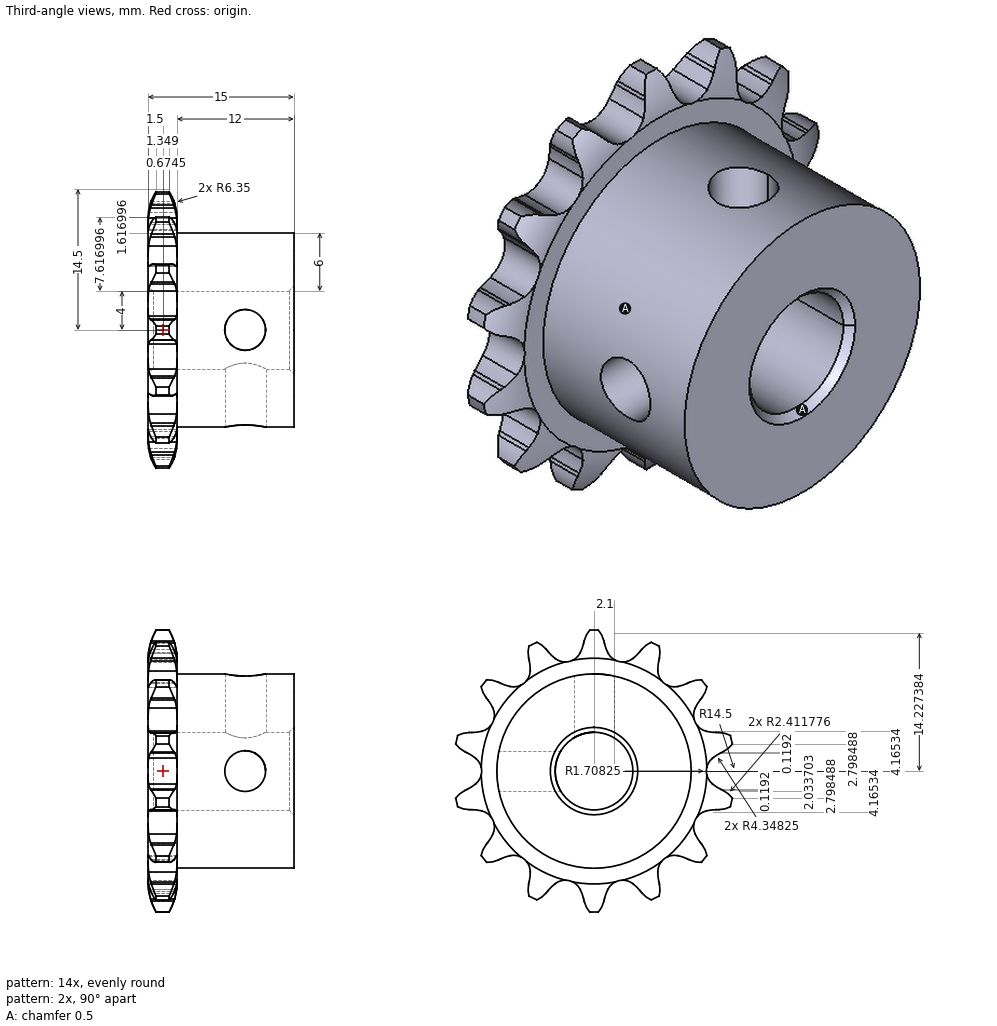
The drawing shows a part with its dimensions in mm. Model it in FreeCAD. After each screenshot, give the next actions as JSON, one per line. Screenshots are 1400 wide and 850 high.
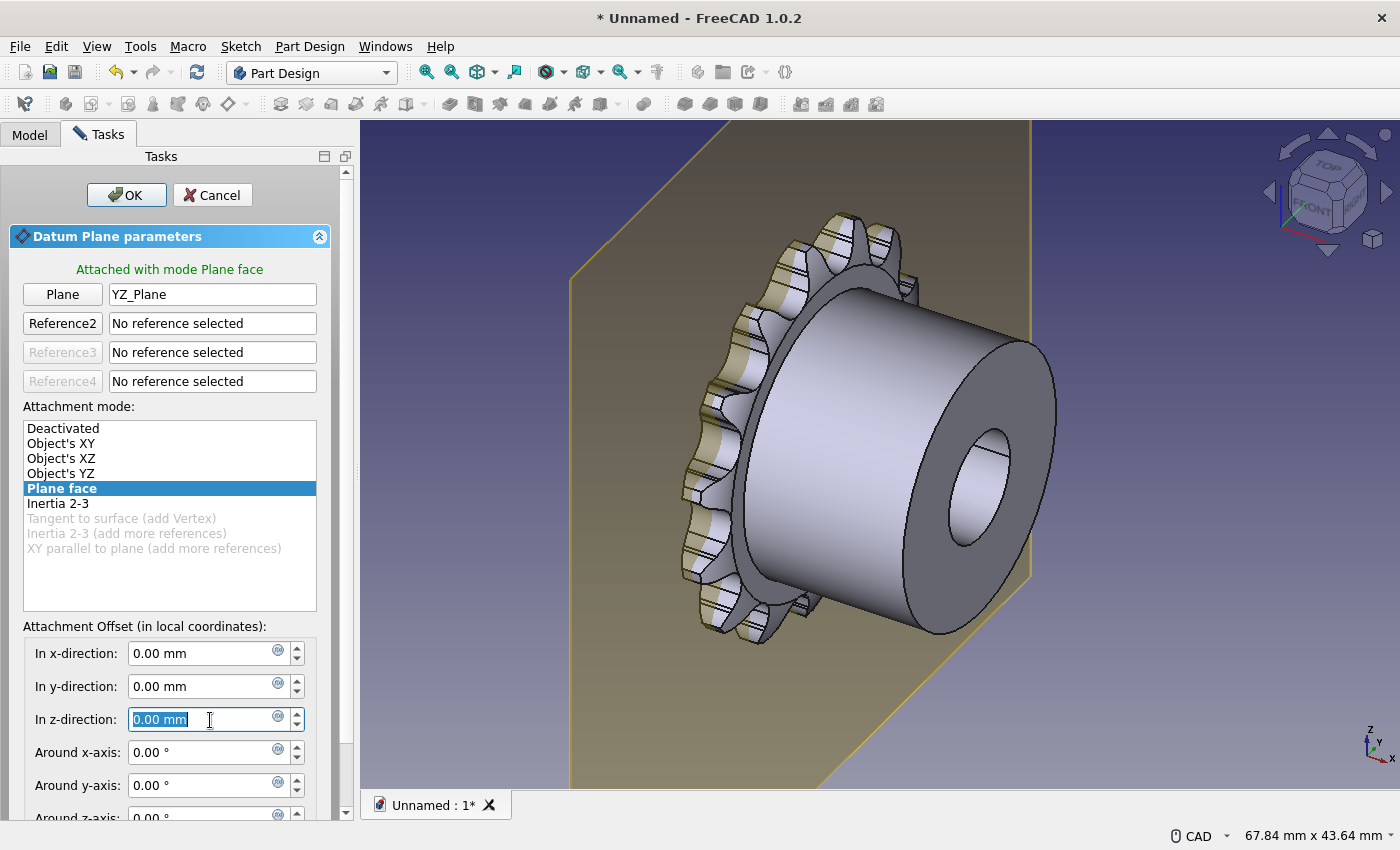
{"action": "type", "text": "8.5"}
{"action": "key", "text": "Tab"}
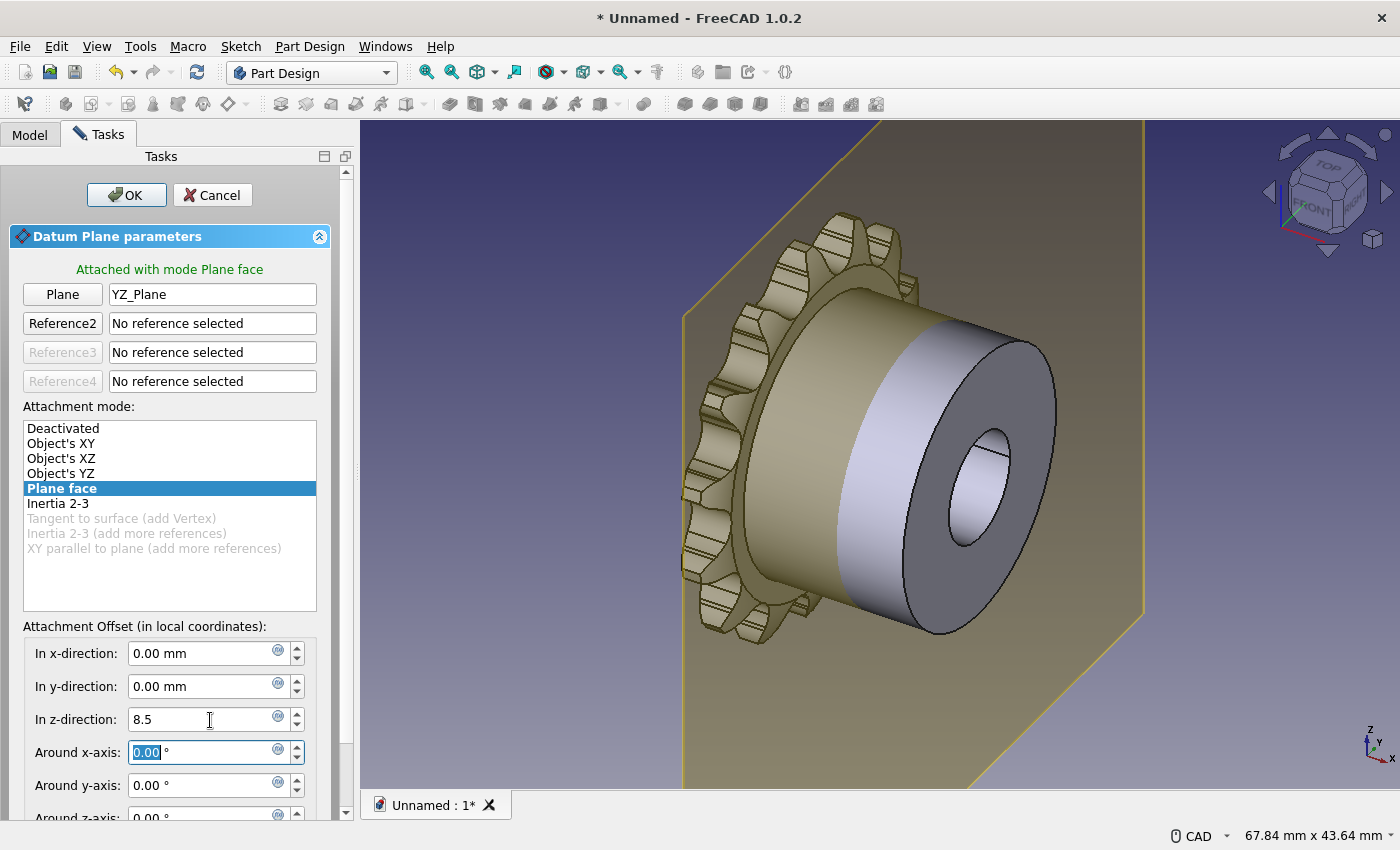
{"action": "left_click", "coordinate": [127, 195]}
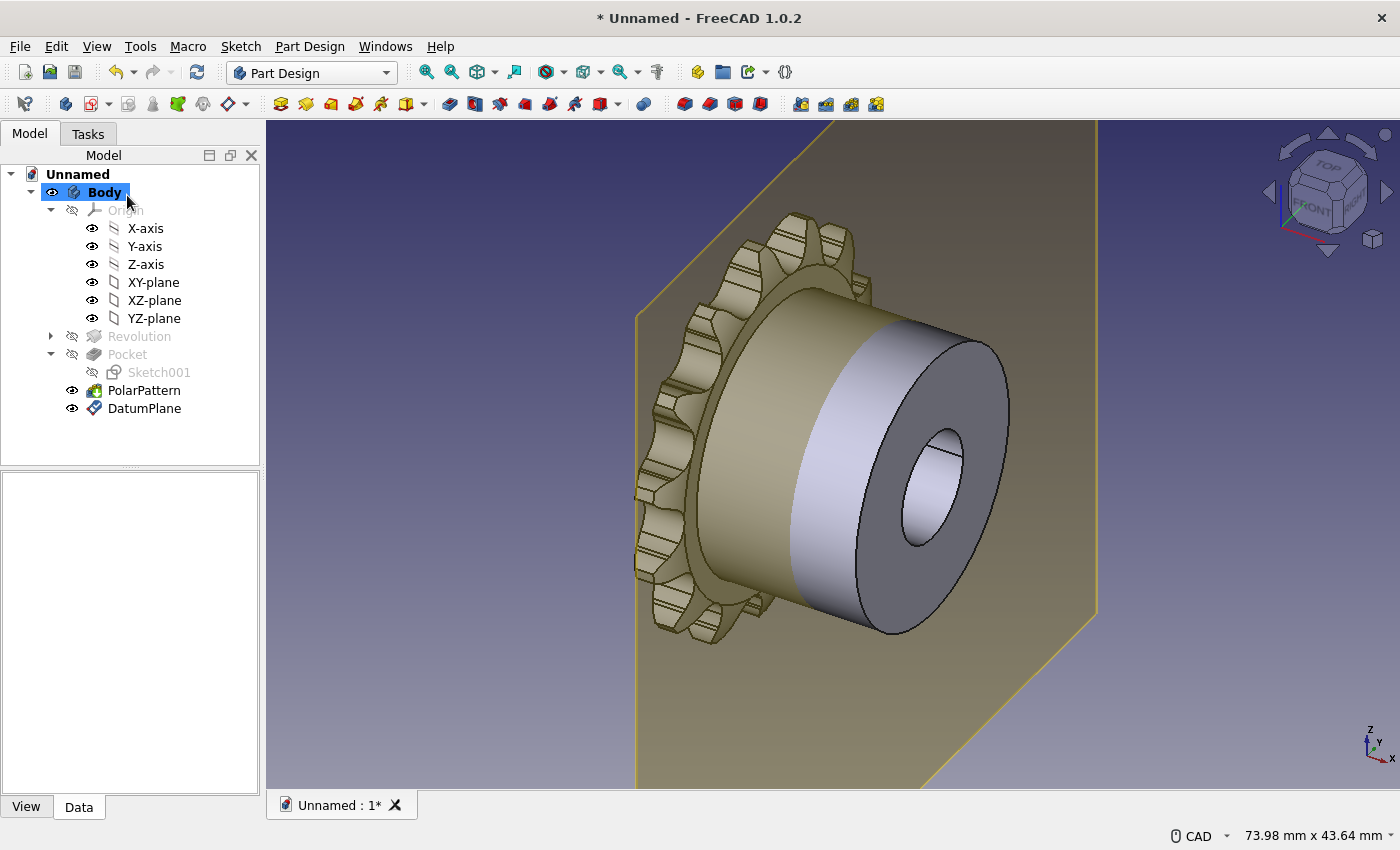
{"action": "left_click", "coordinate": [117, 408]}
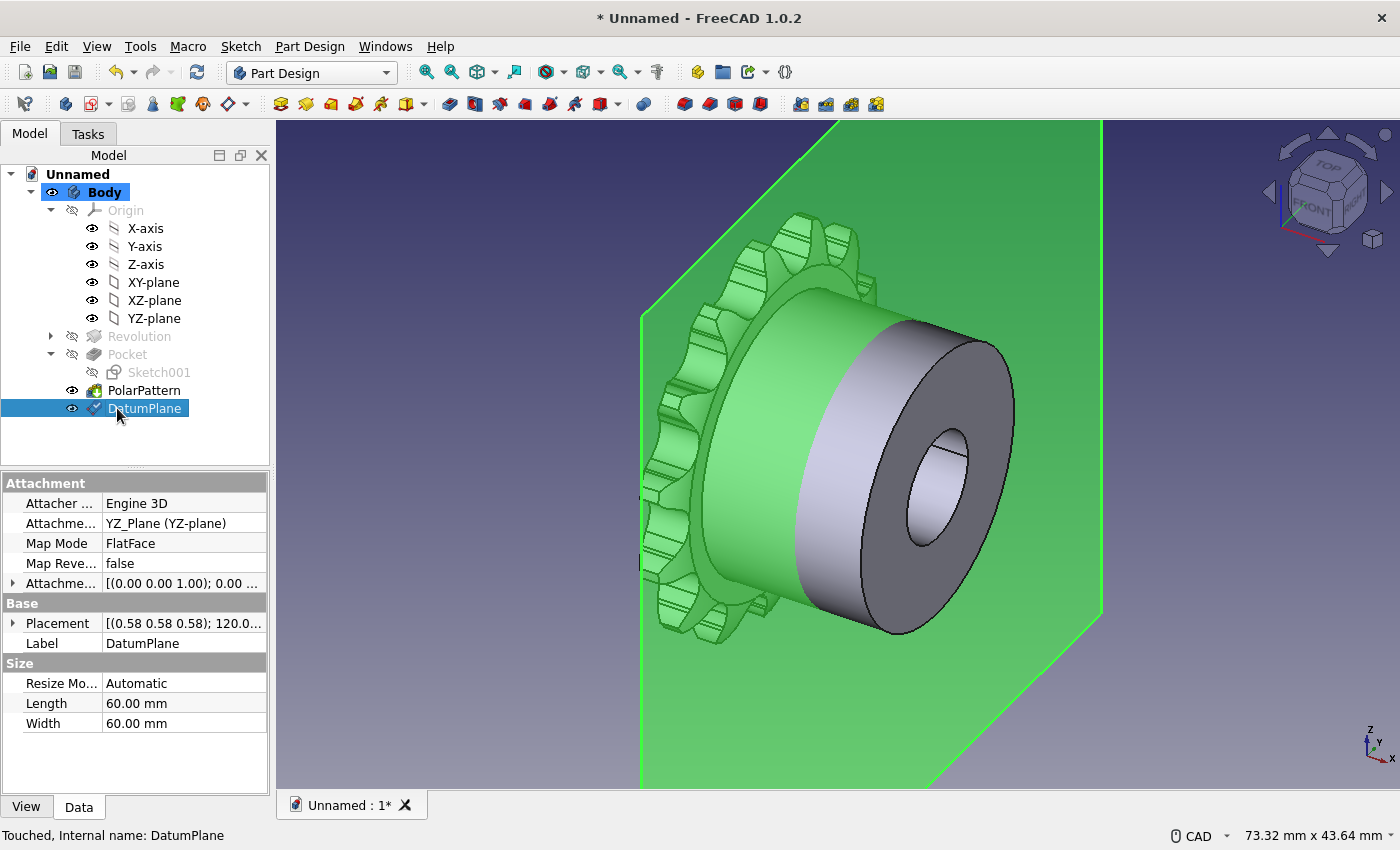
{"action": "left_click", "coordinate": [90, 104]}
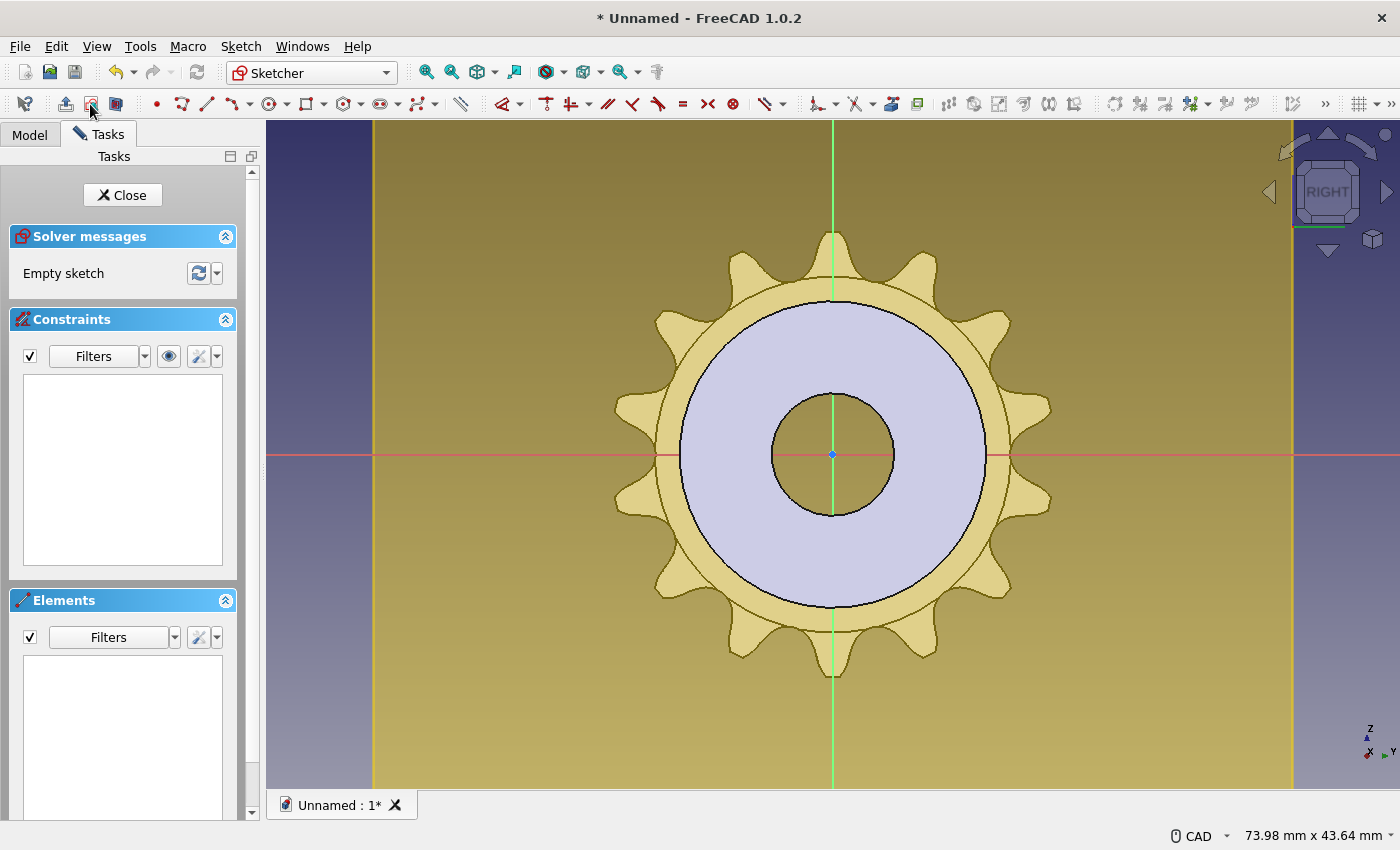
{"action": "left_click", "coordinate": [116, 104]}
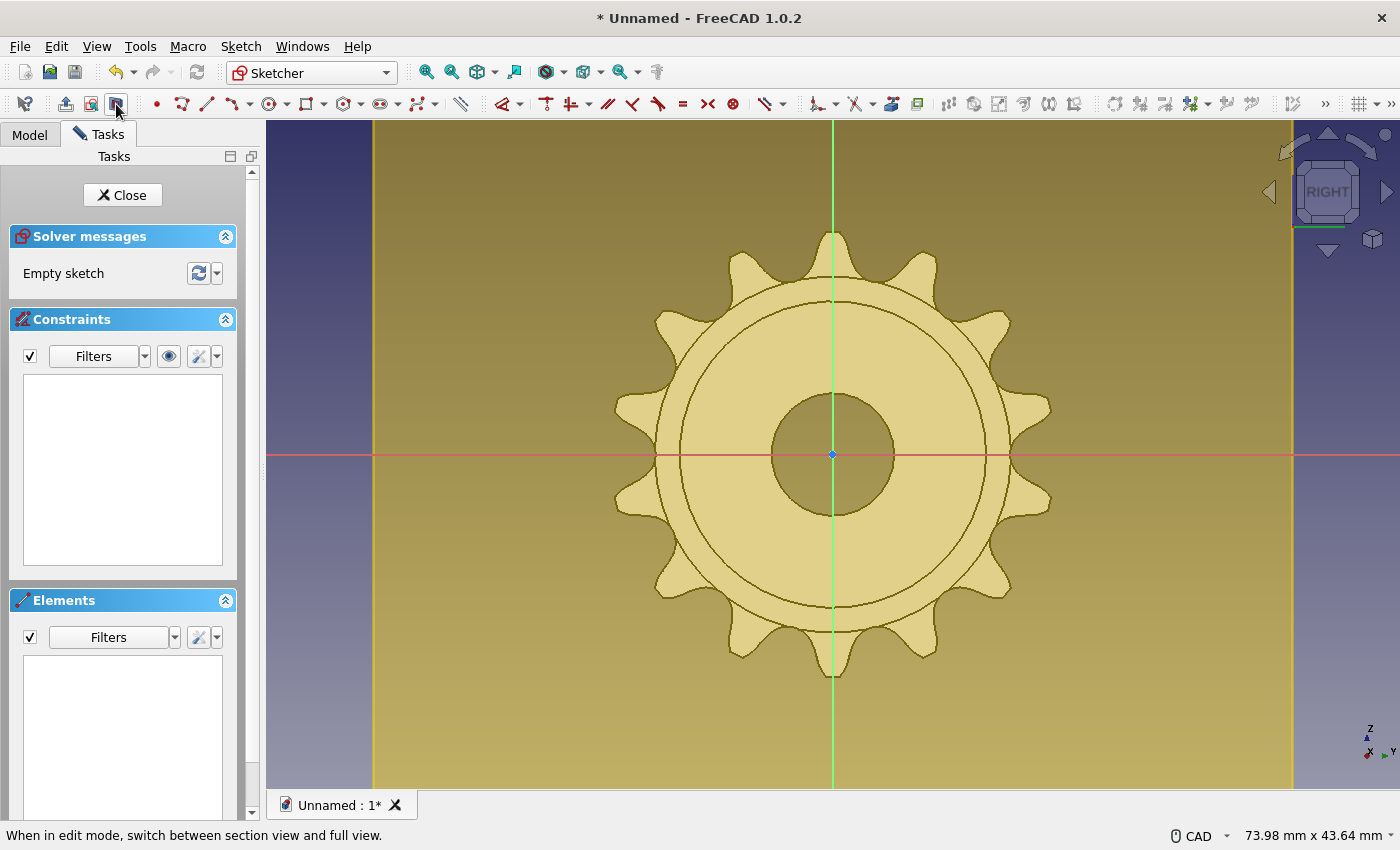
{"action": "scroll", "coordinate": [952, 213], "scroll_direction": "up", "scroll_amount": 3}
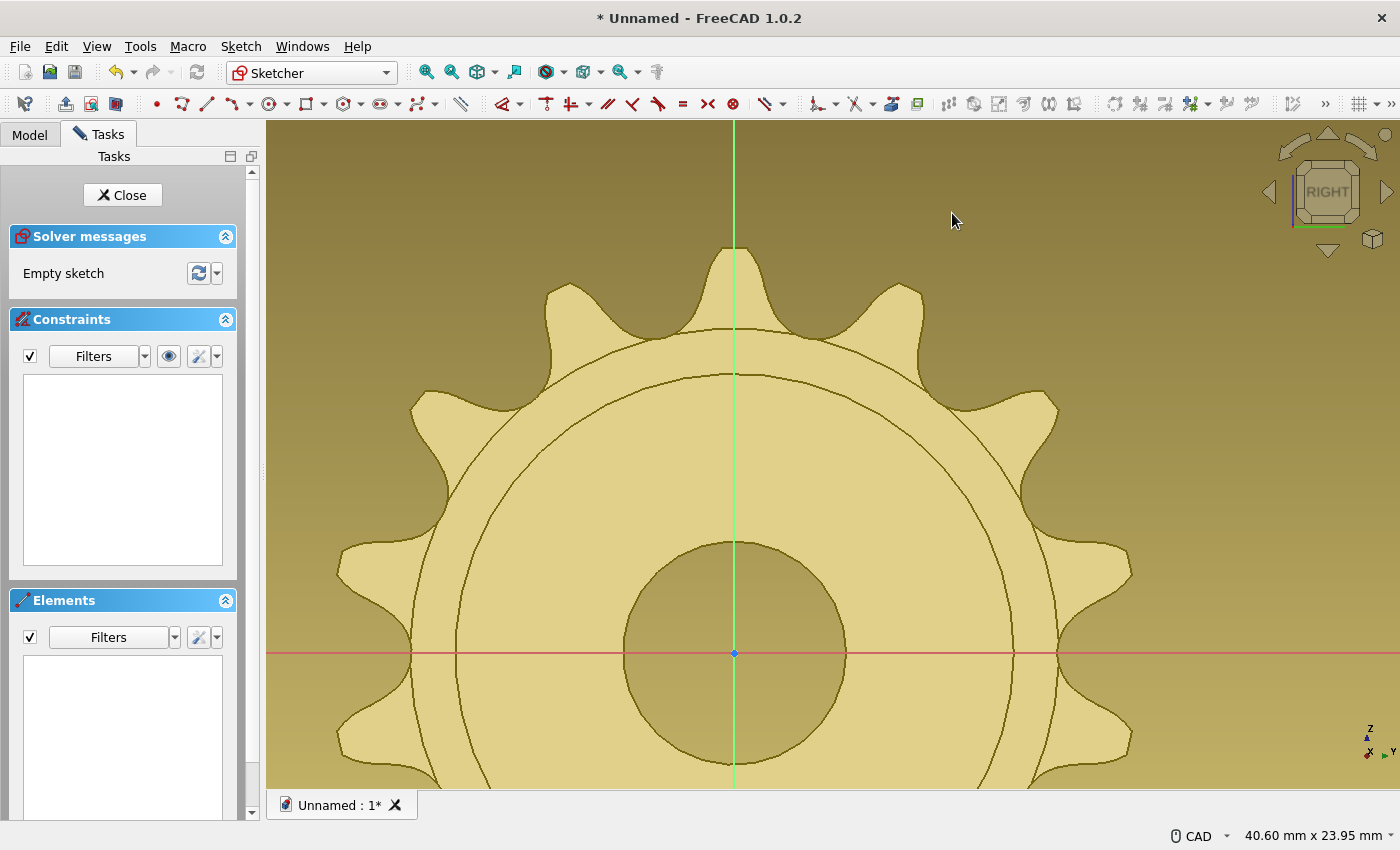
{"action": "left_click", "coordinate": [306, 104]}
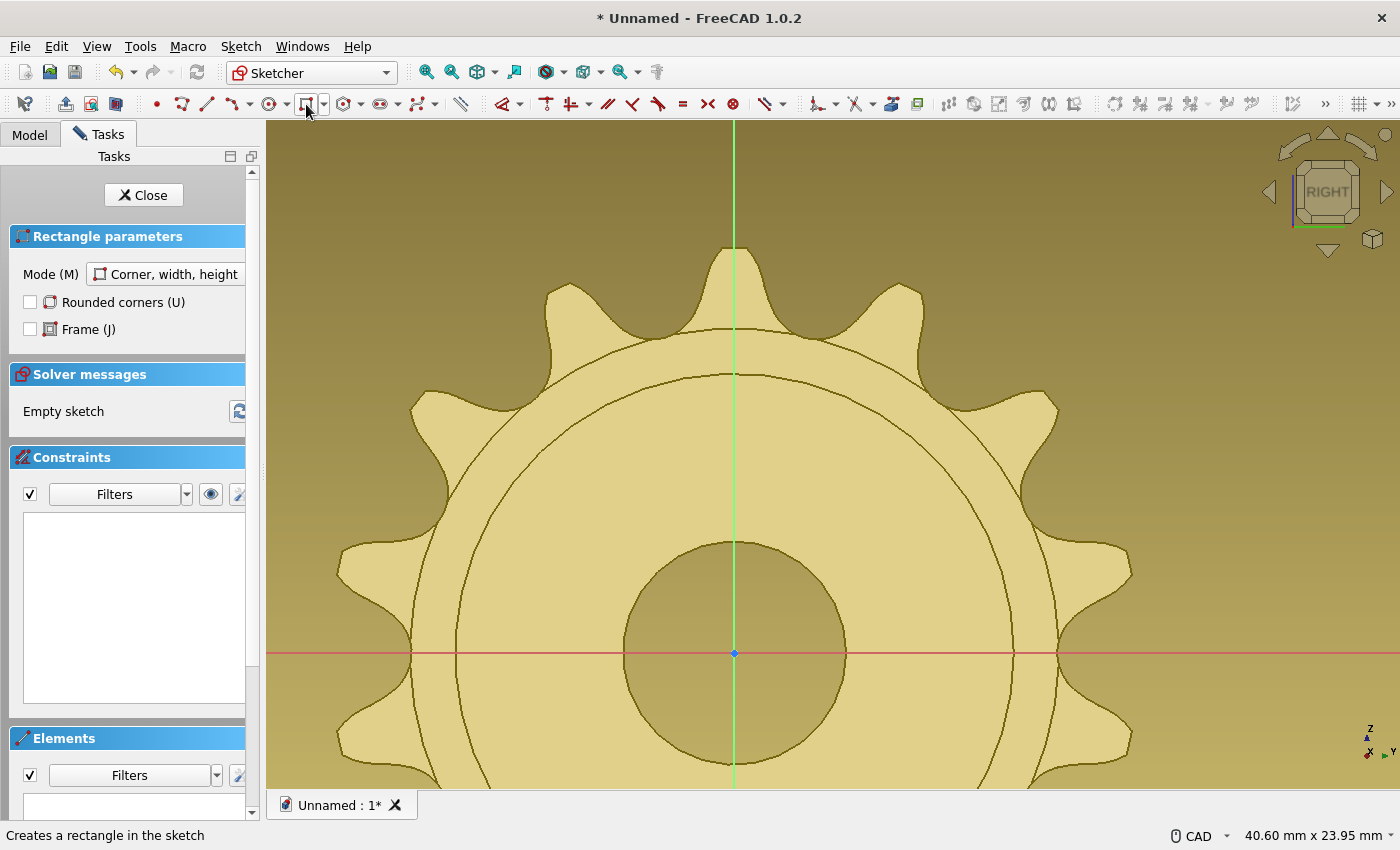
{"action": "left_click", "coordinate": [734, 653]}
{"action": "left_click", "coordinate": [793, 256]}
{"action": "key", "text": "Escape"}